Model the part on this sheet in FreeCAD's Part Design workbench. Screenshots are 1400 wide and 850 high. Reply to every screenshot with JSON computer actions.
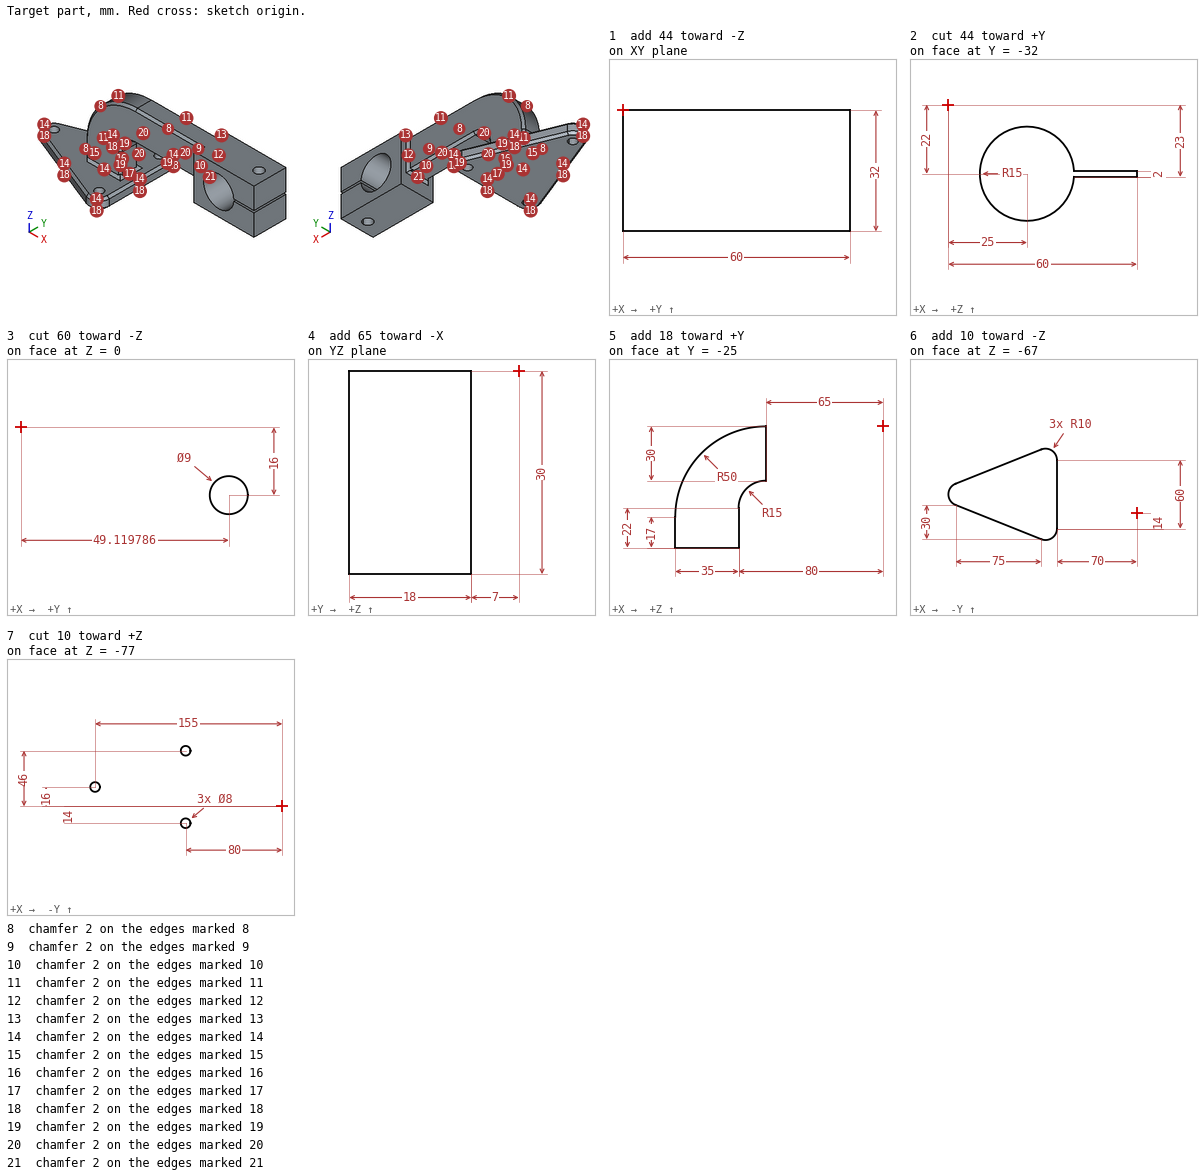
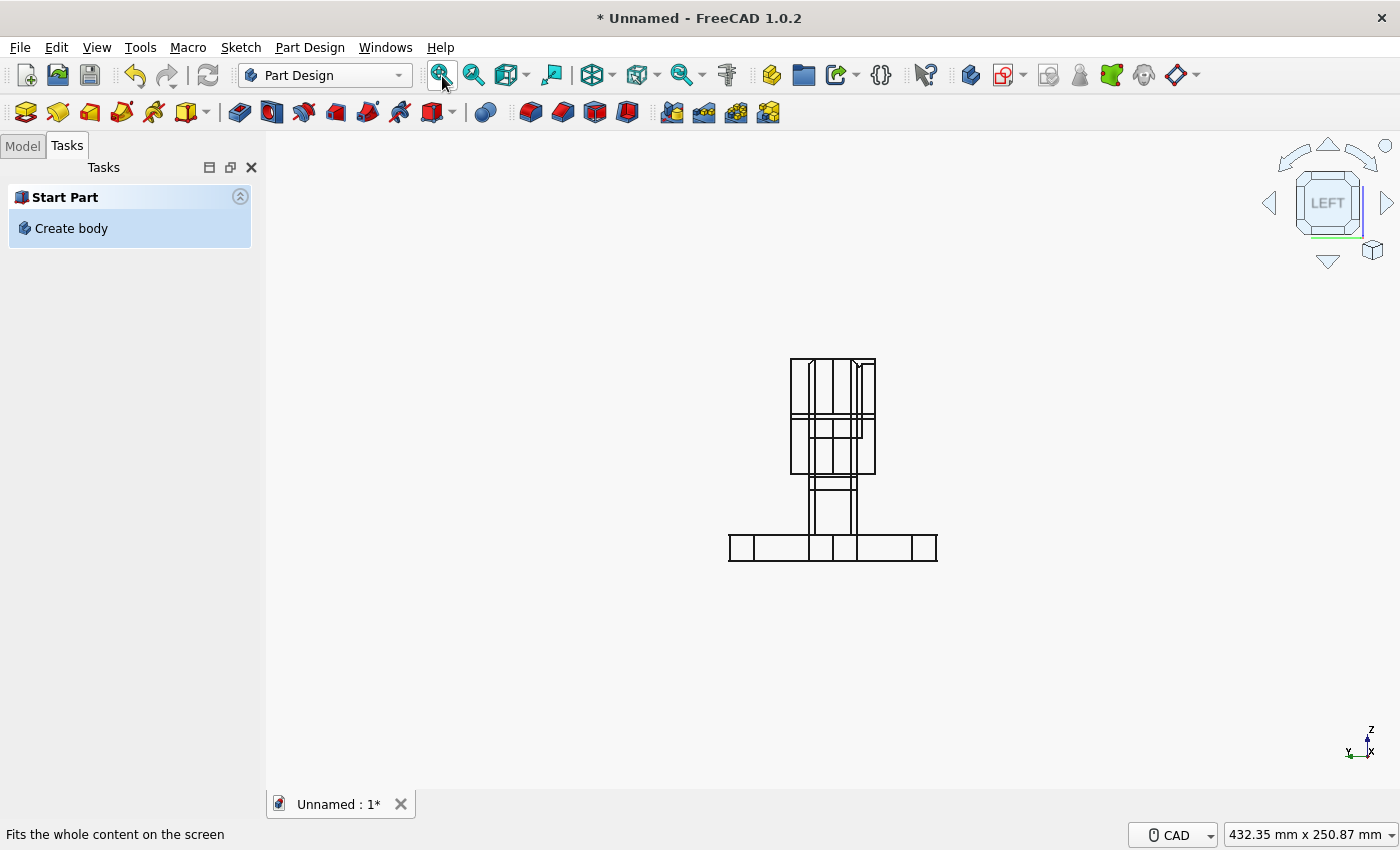
{"action": "key", "text": "0"}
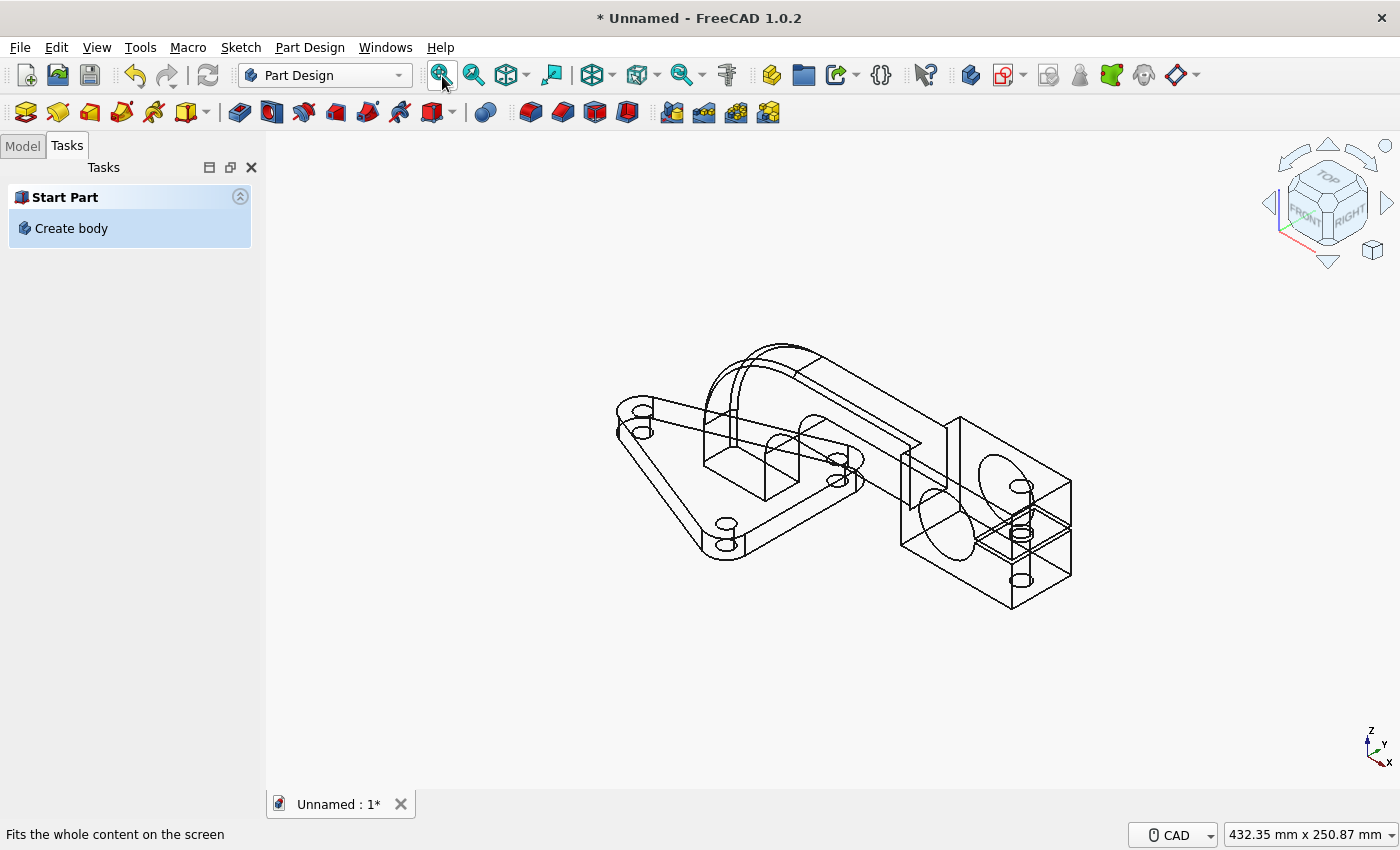
{"action": "left_click", "coordinate": [947, 457]}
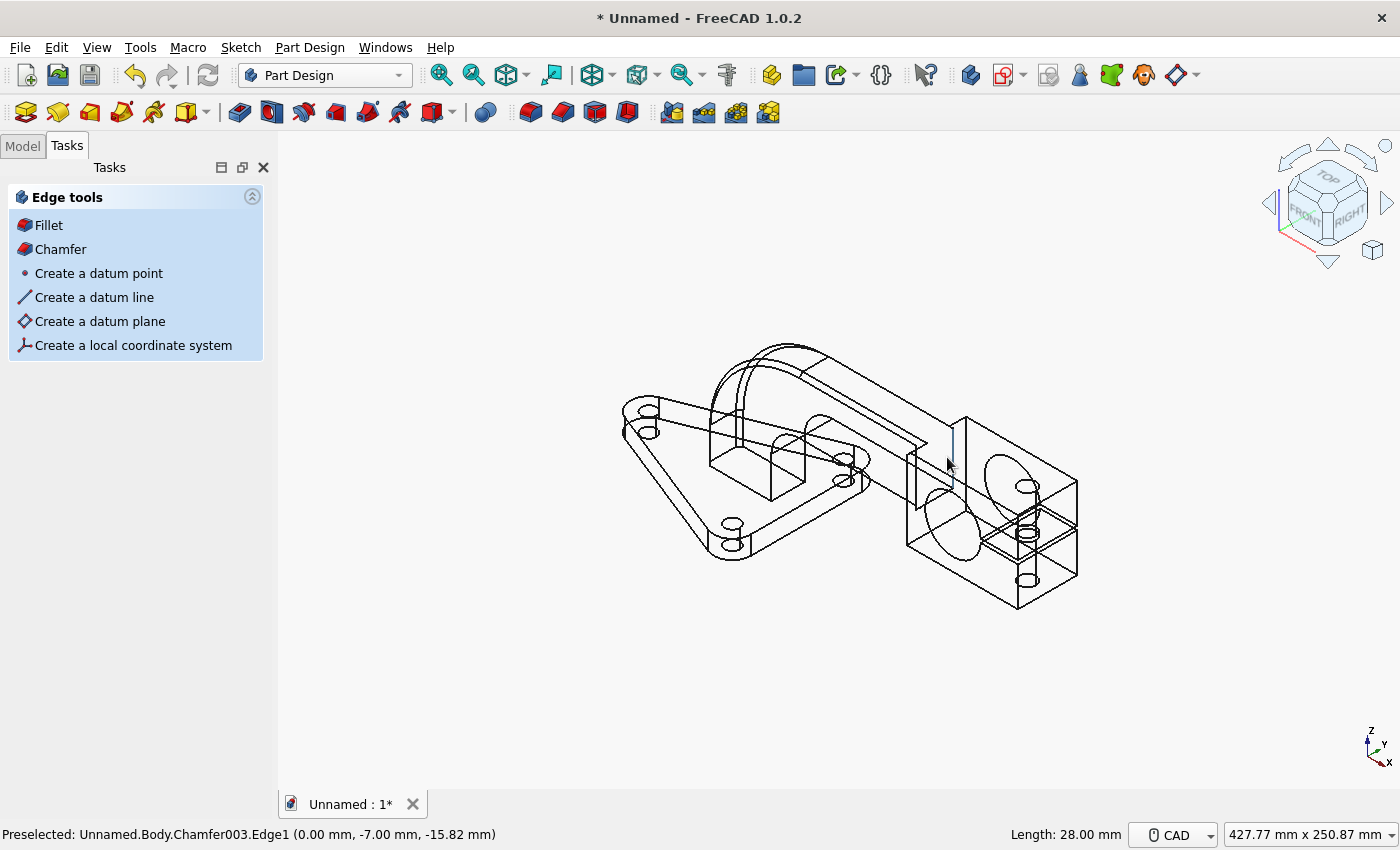
{"action": "key", "text": "v 1"}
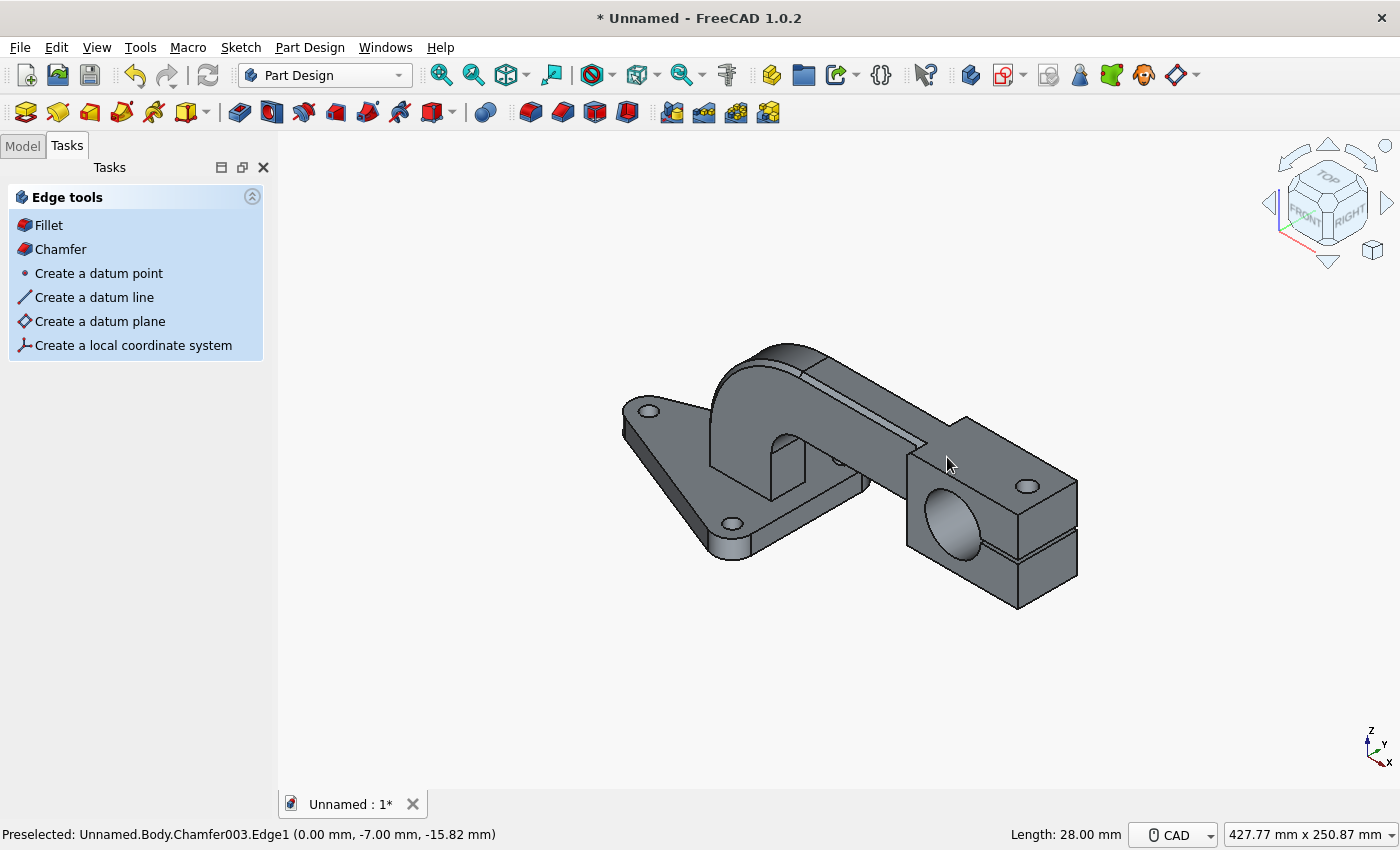
{"action": "left_click", "coordinate": [564, 112]}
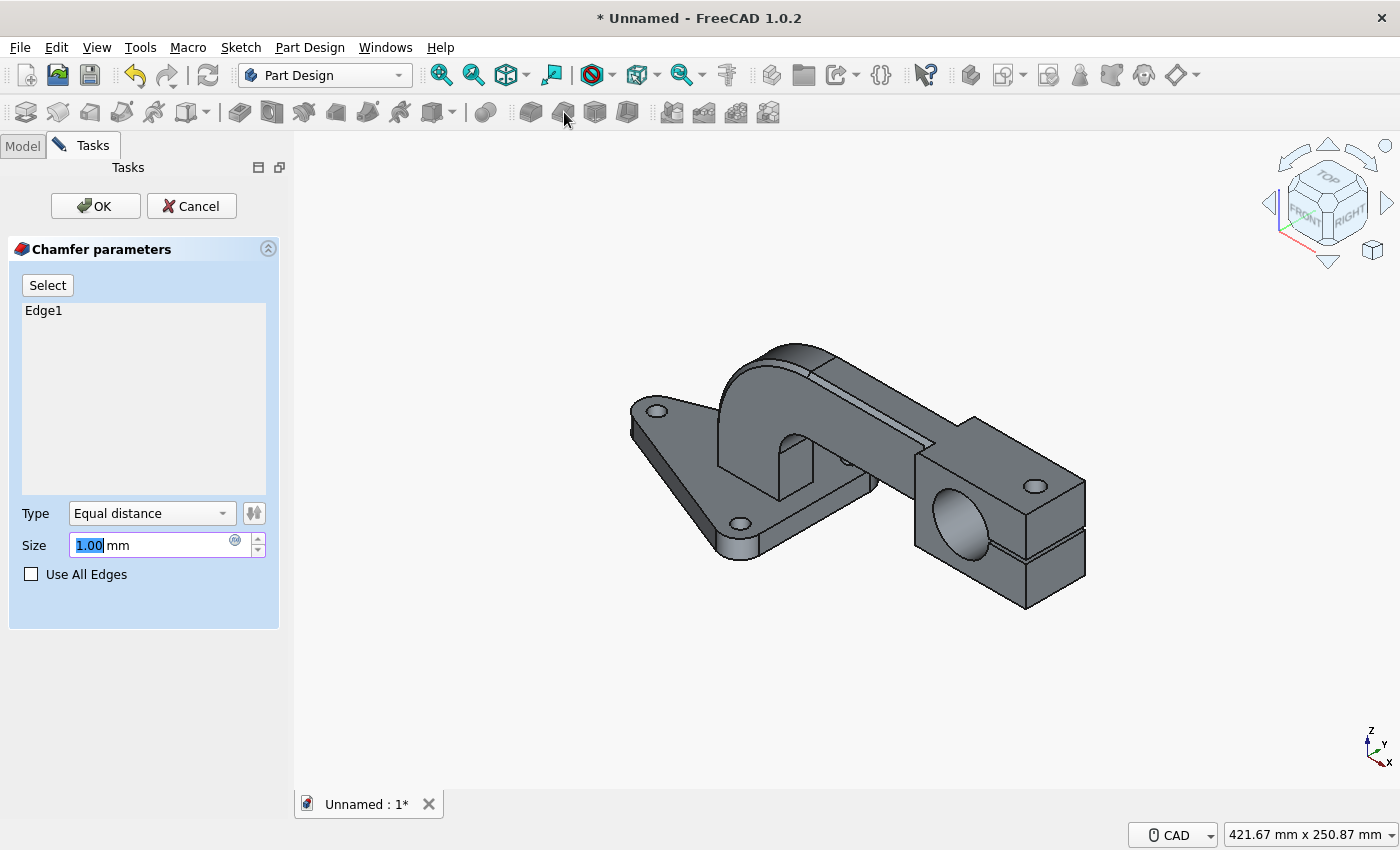
{"action": "type", "text": "2"}
{"action": "key", "text": "Tab"}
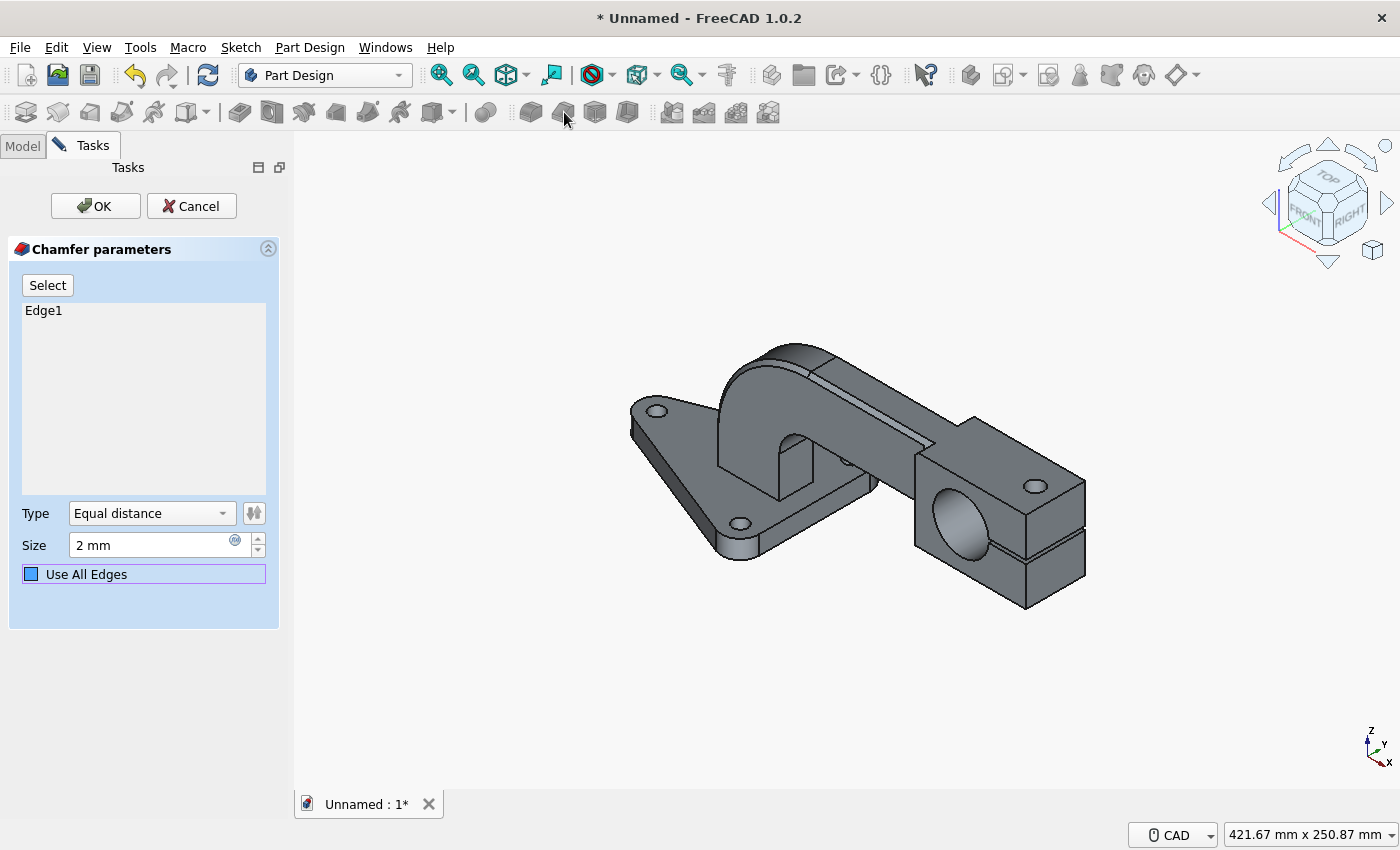
{"action": "left_click", "coordinate": [96, 206]}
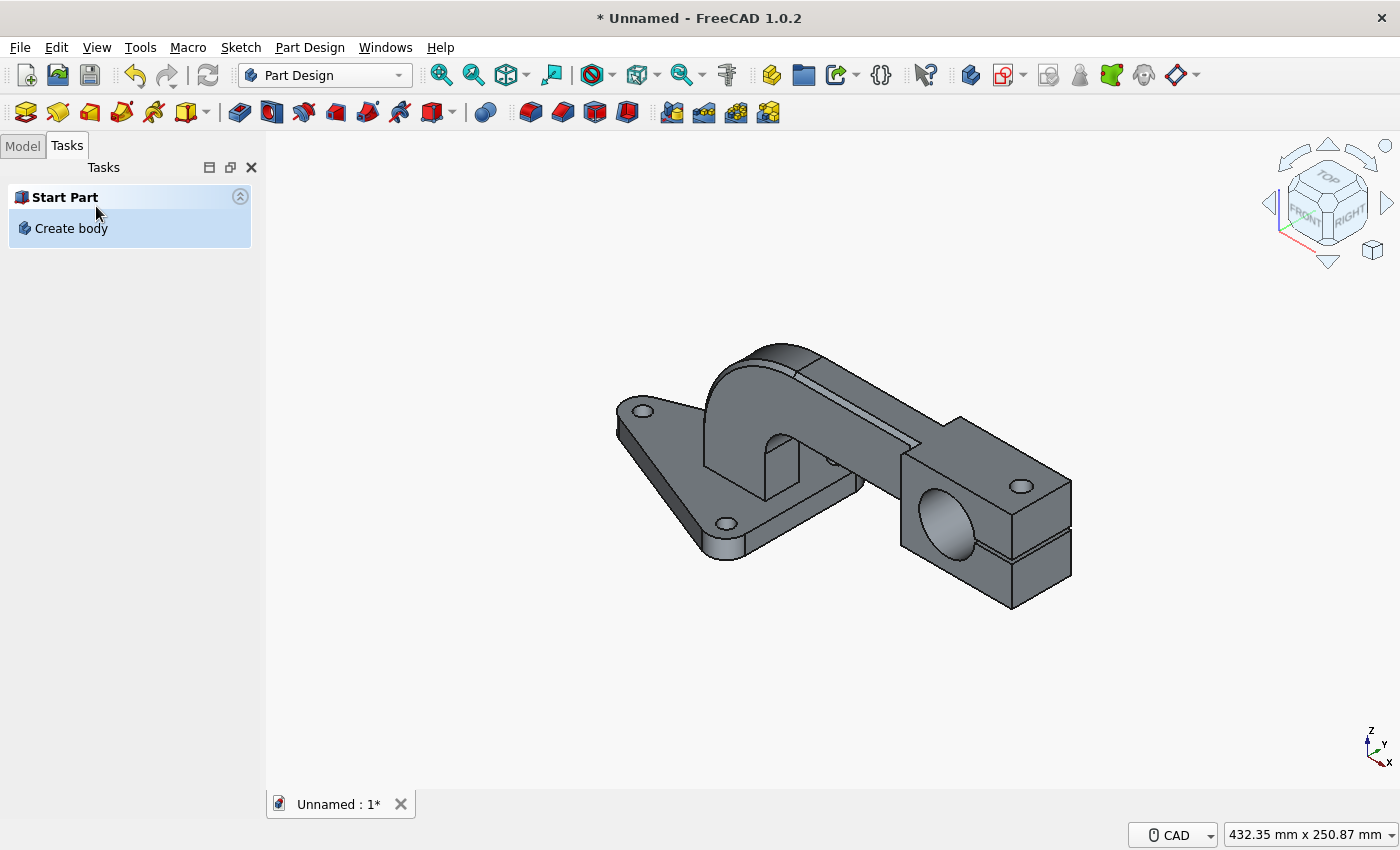
{"action": "scroll", "coordinate": [954, 419], "scroll_direction": "up", "scroll_amount": 4}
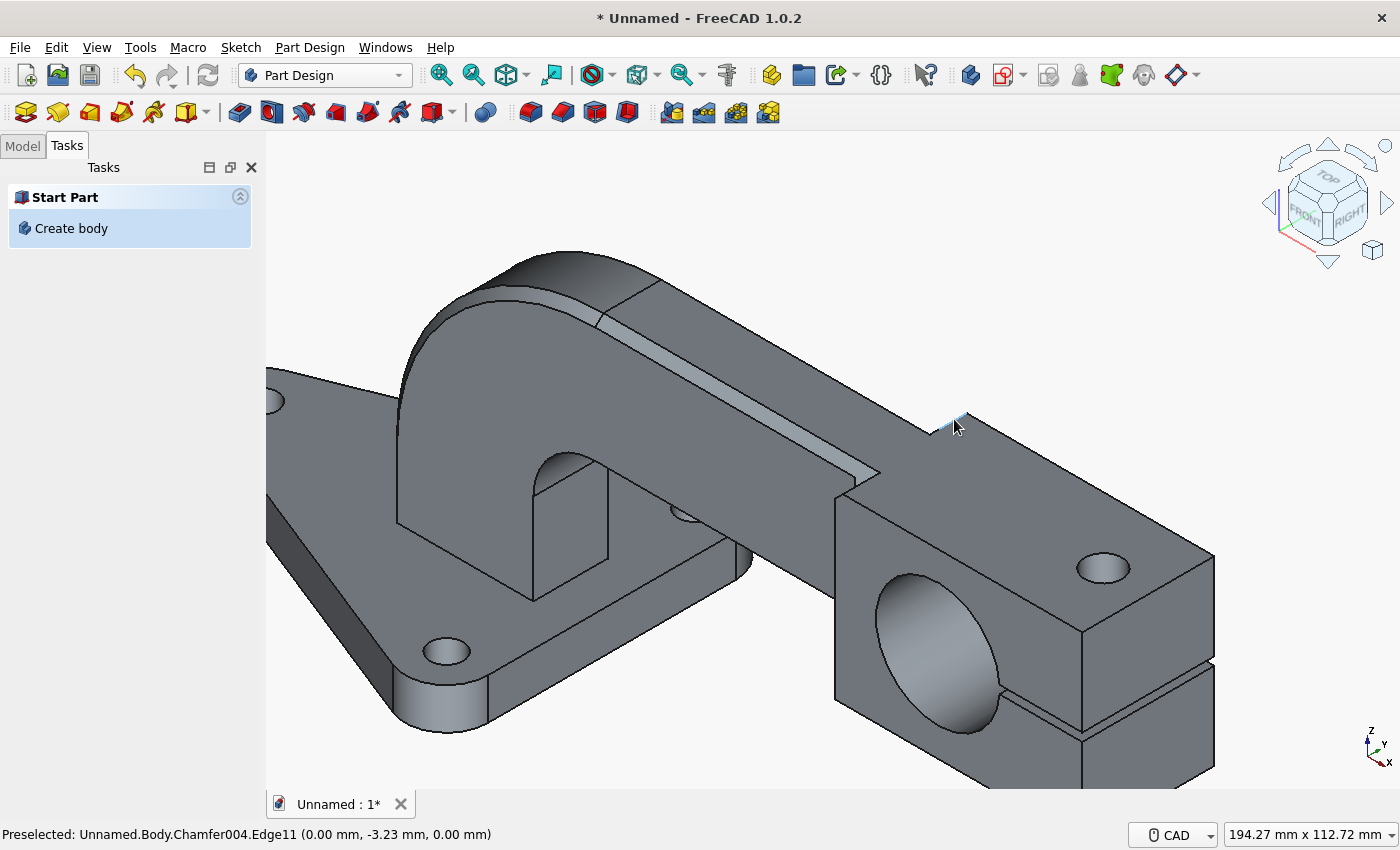
{"action": "left_click", "coordinate": [442, 76]}